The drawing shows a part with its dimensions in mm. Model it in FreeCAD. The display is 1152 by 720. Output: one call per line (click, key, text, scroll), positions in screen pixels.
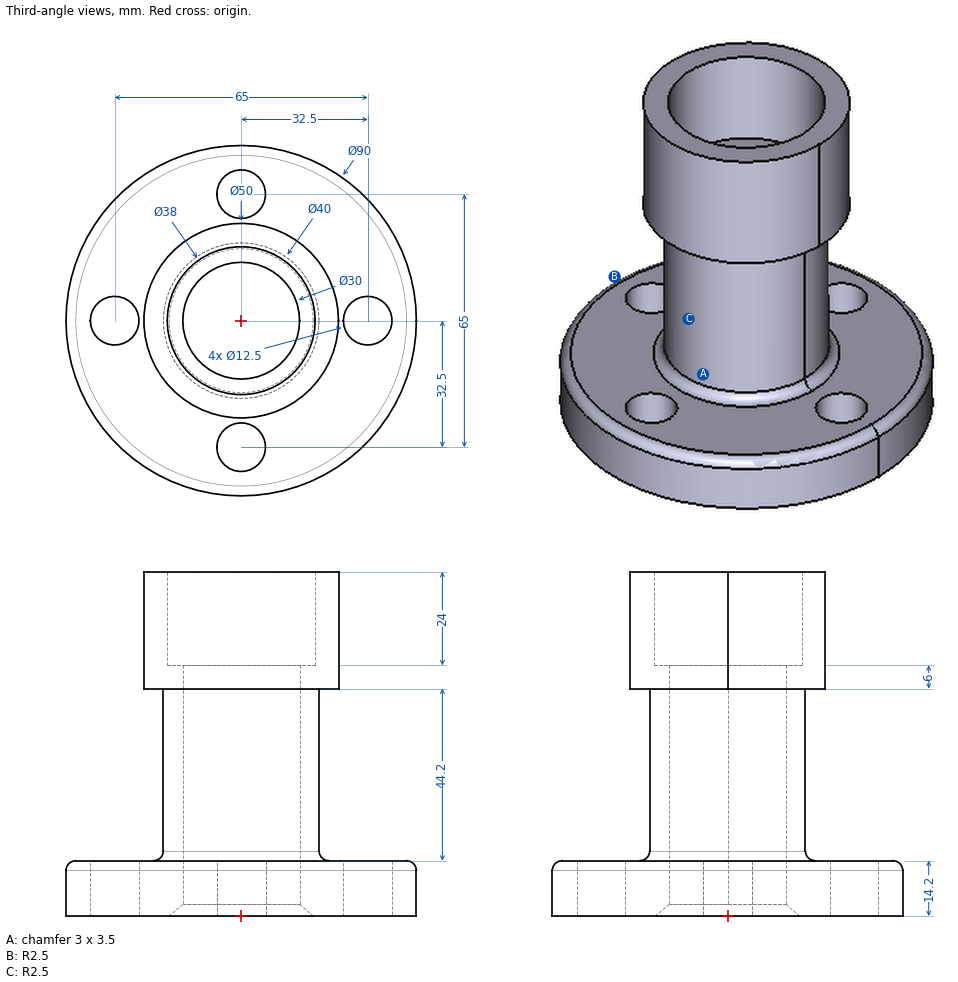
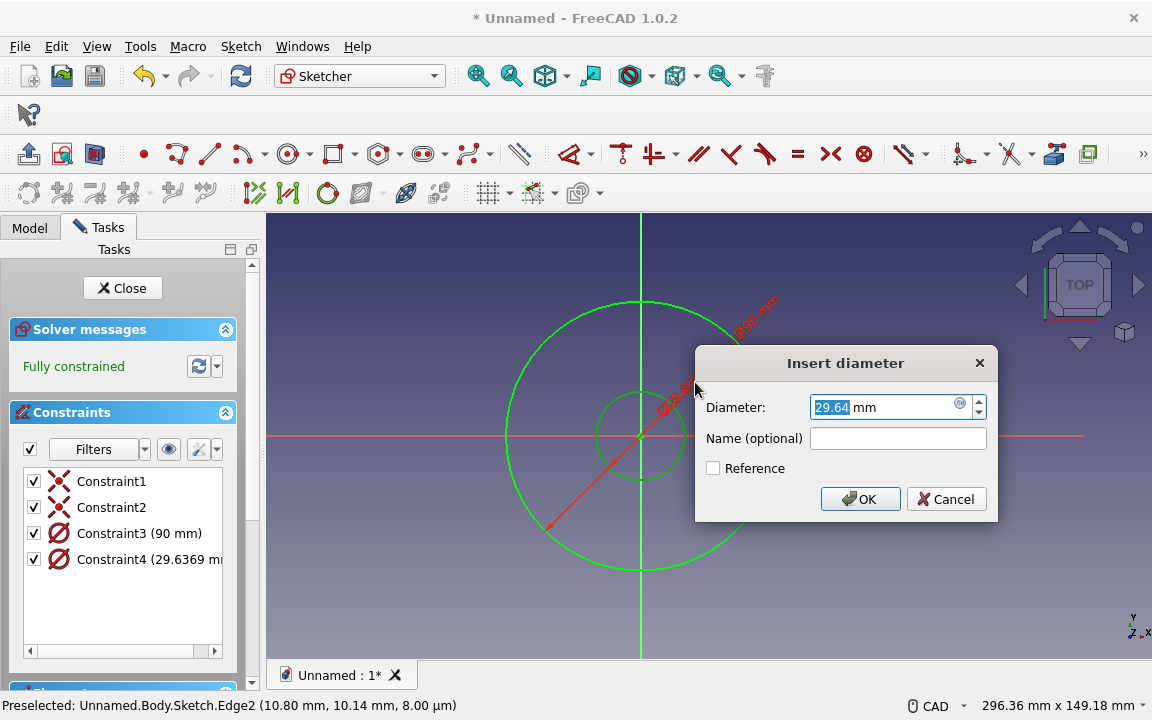
text(30)
key(Return)
key(Escape)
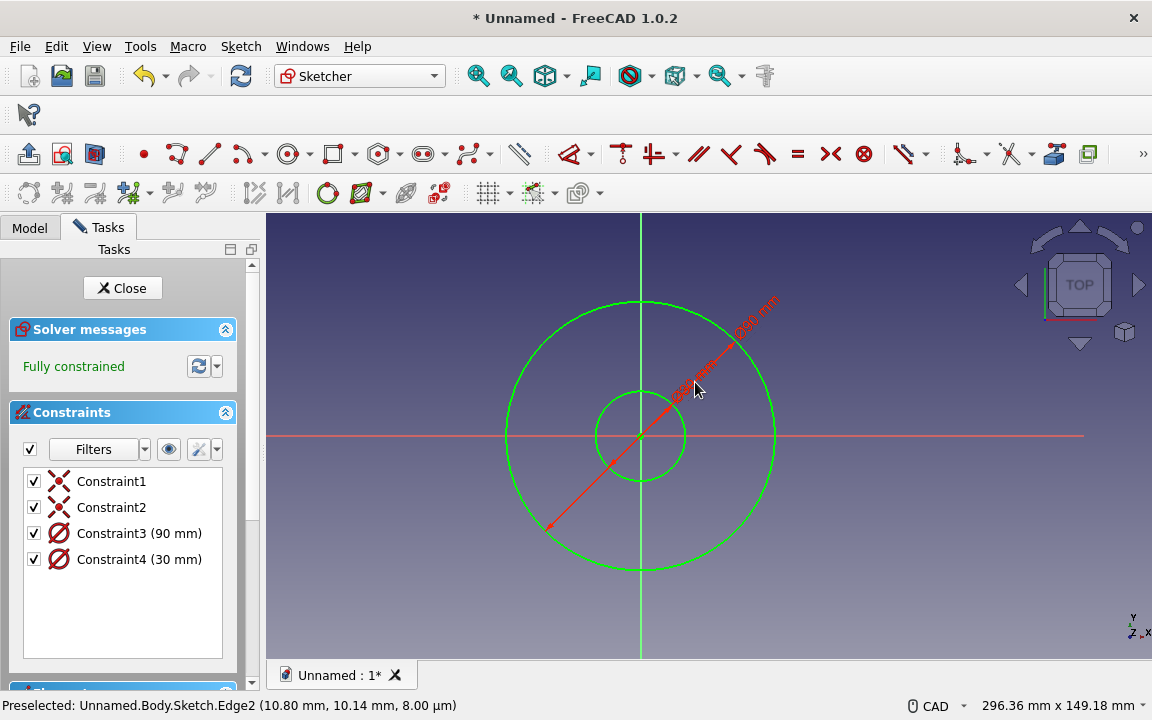
click(123, 288)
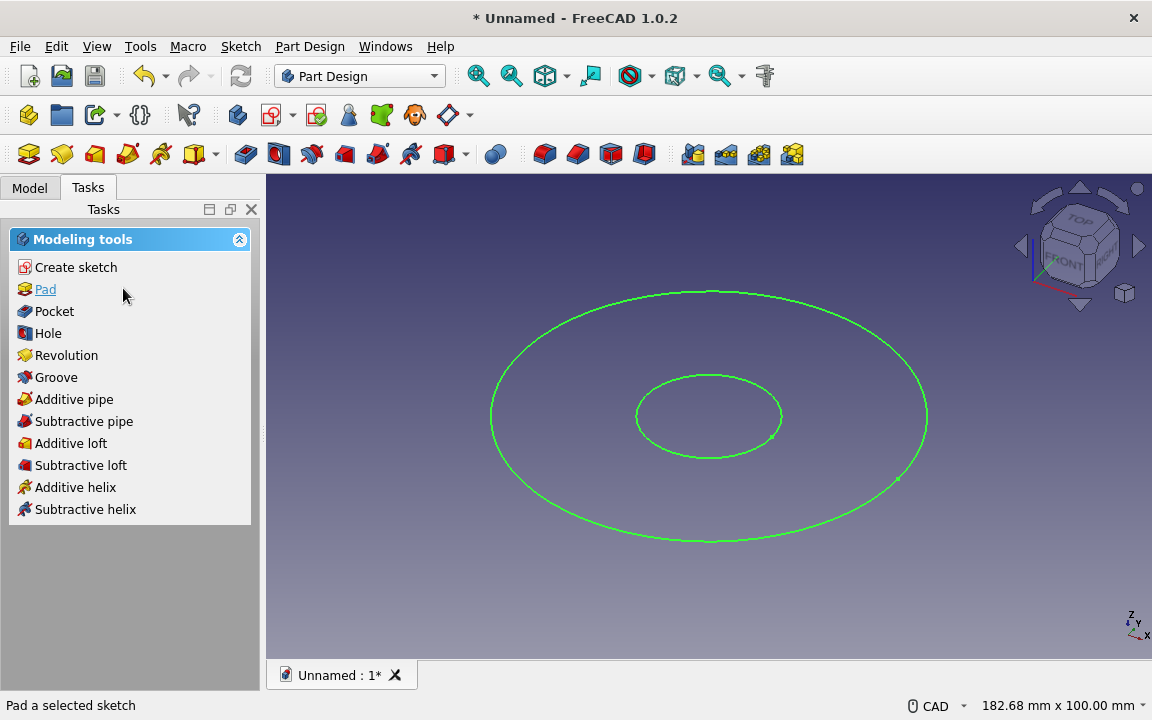
click(29, 154)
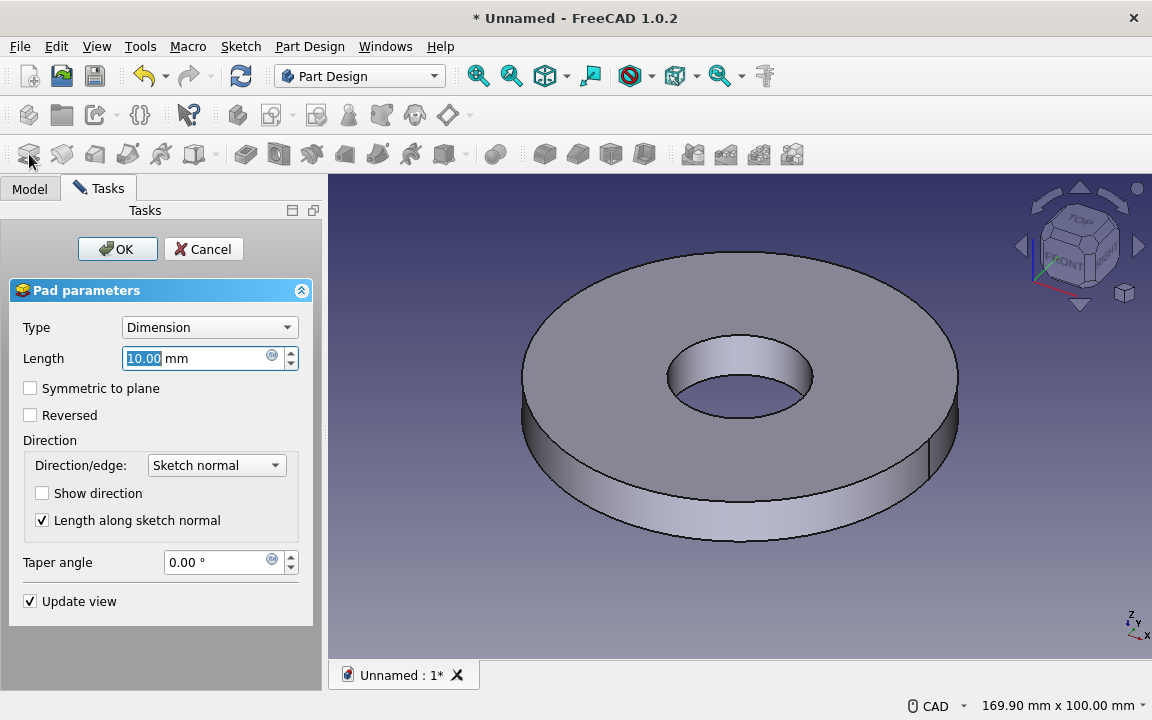
text(14.2)
key(Tab)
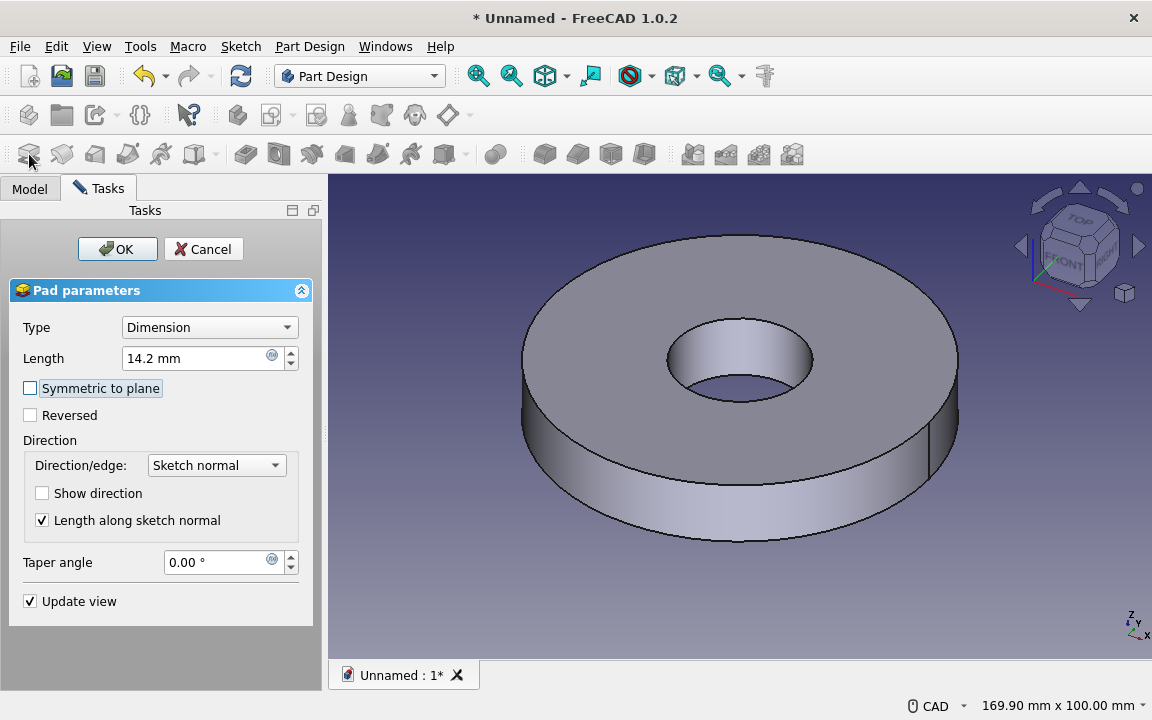
click(118, 249)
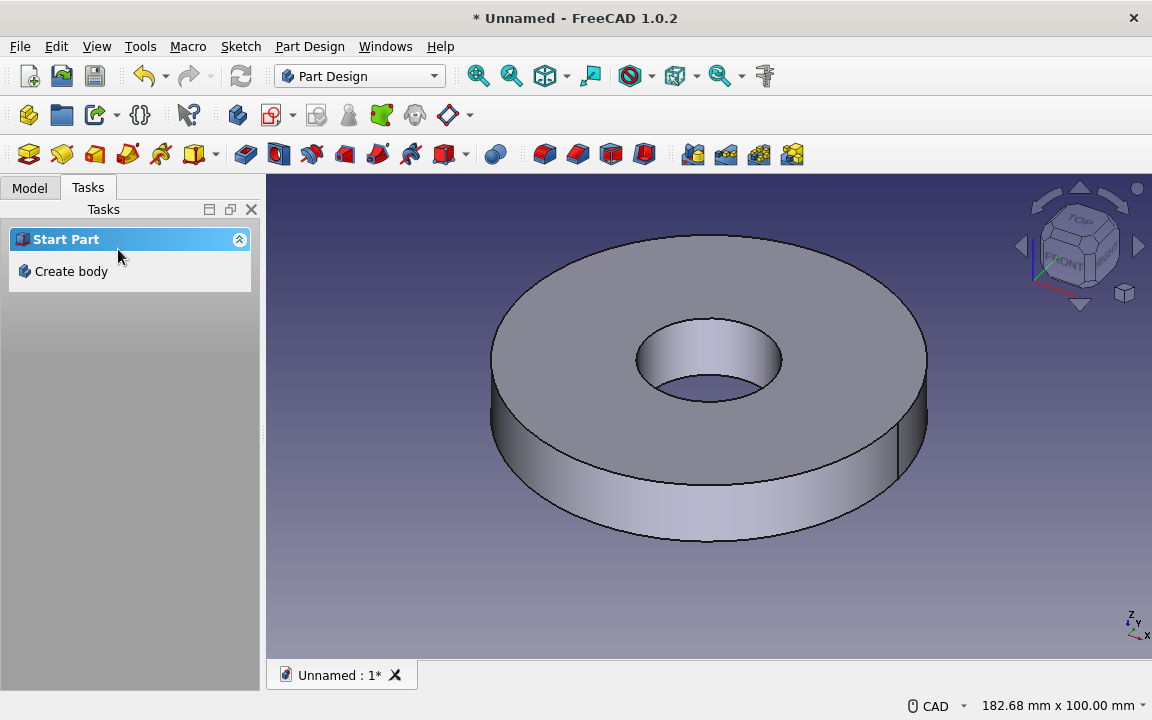
key(5)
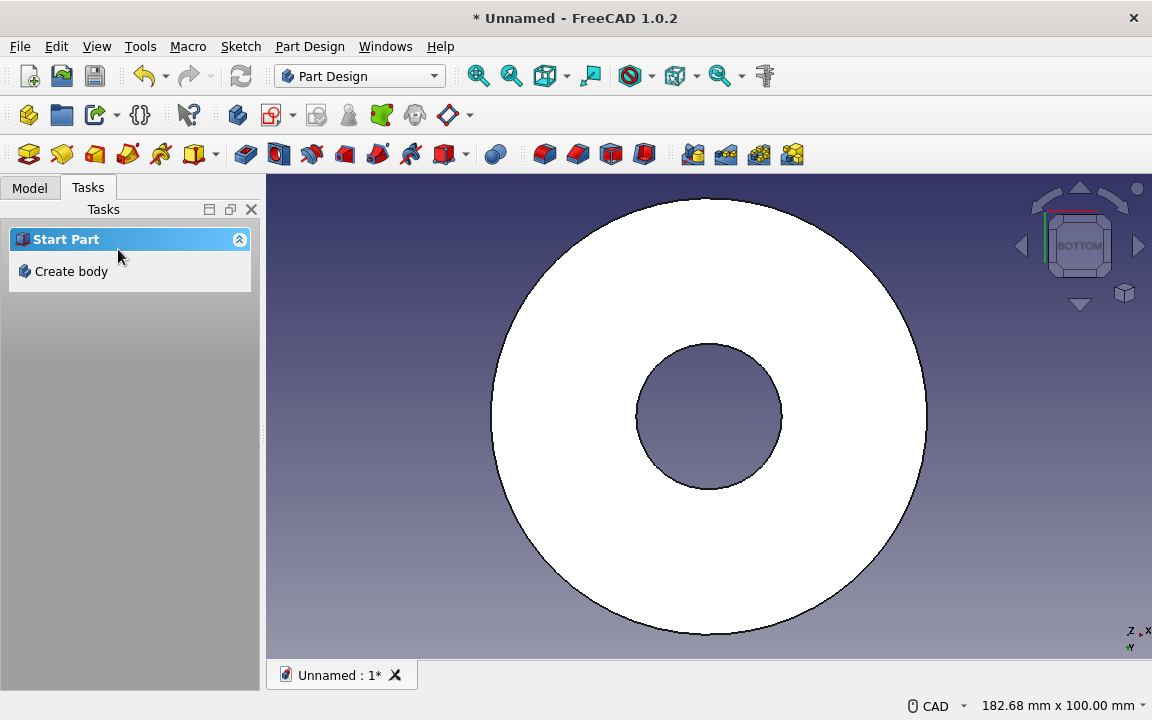
click(647, 291)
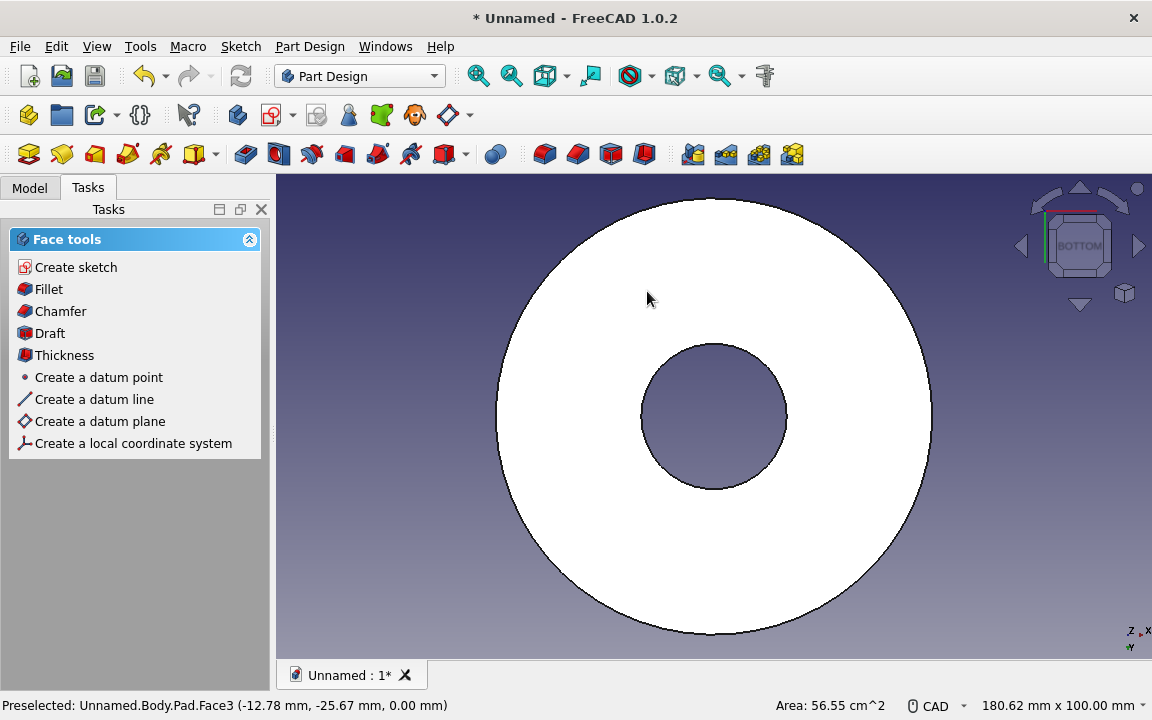
click(270, 116)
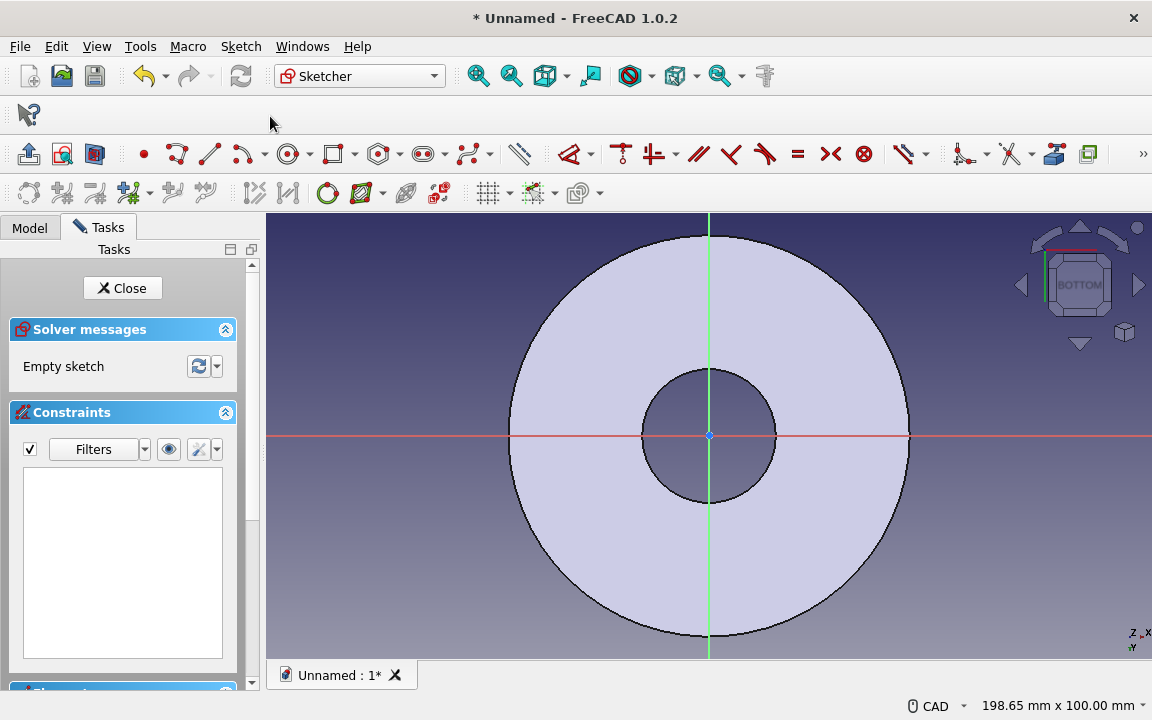
scroll(331, 436, down, 1)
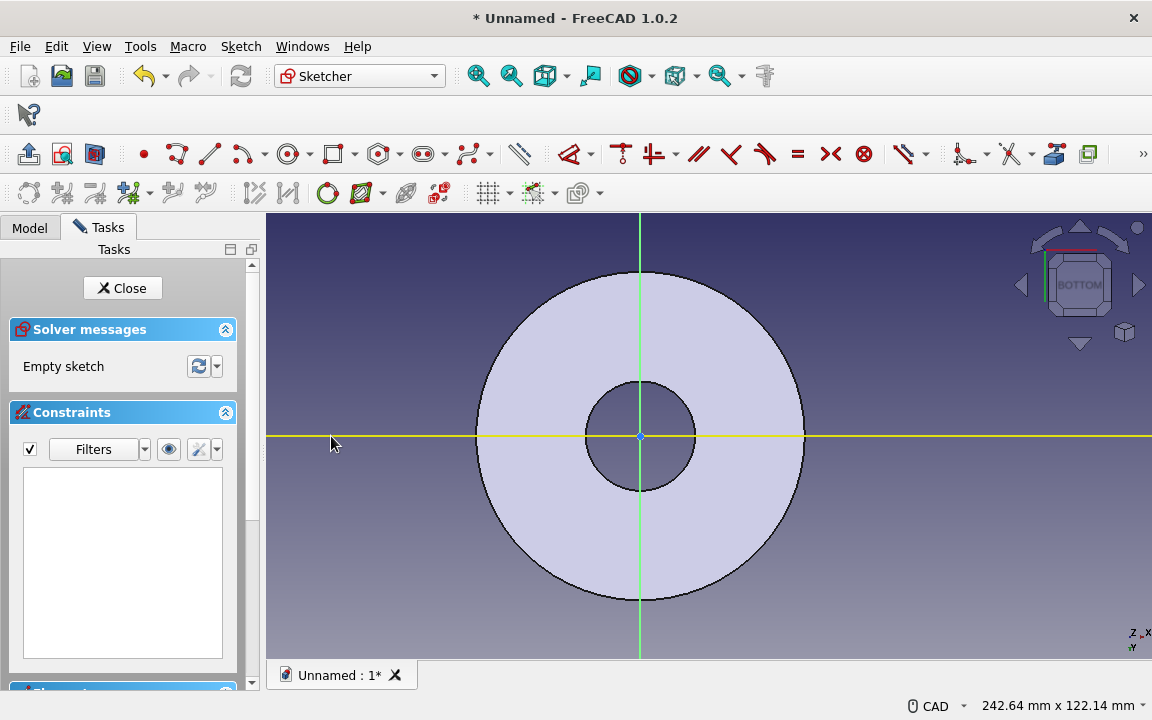
click(288, 154)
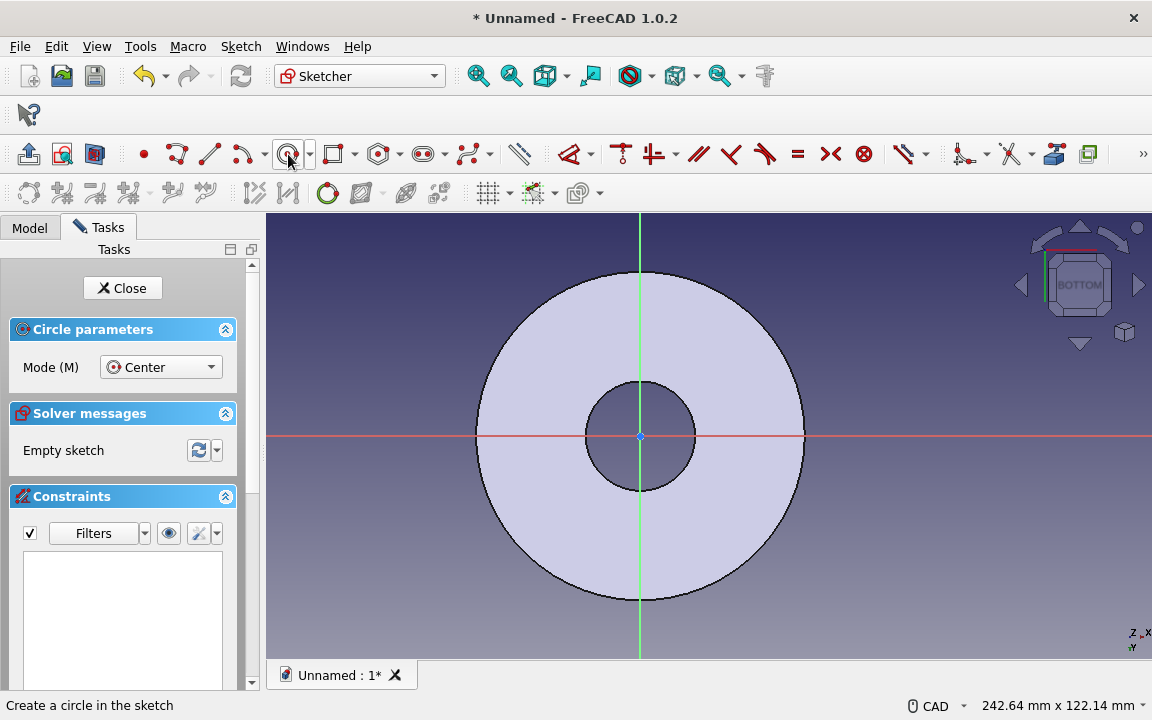
click(759, 436)
click(775, 420)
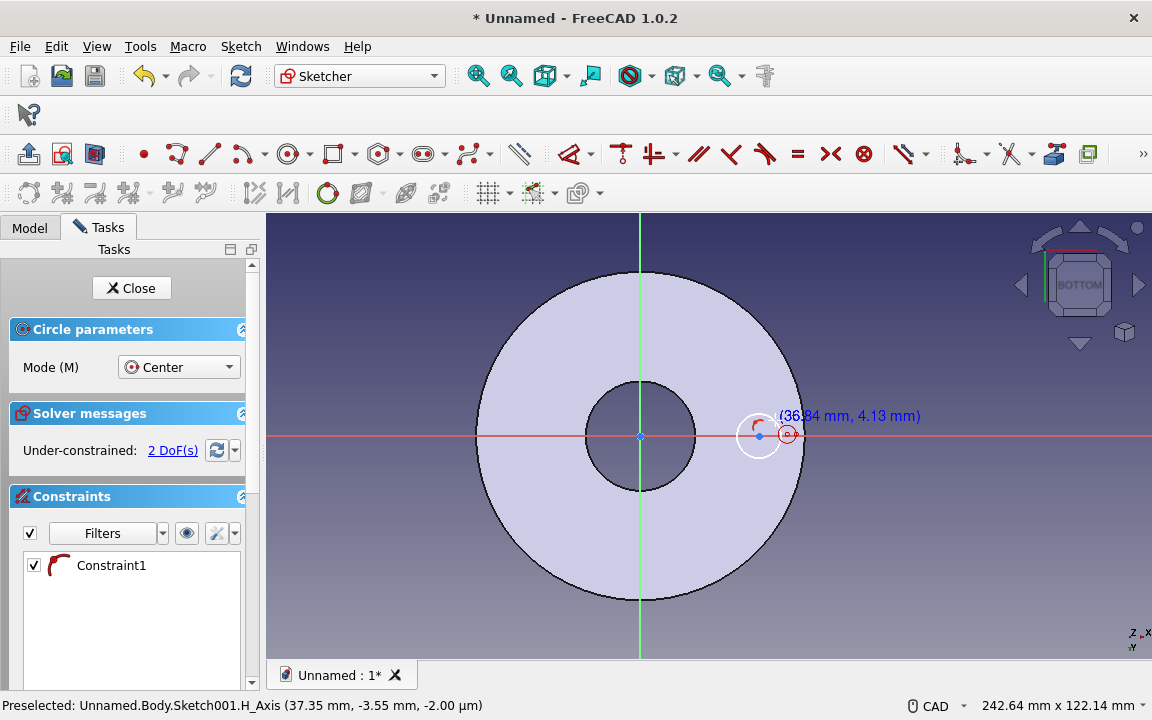
click(522, 436)
click(538, 420)